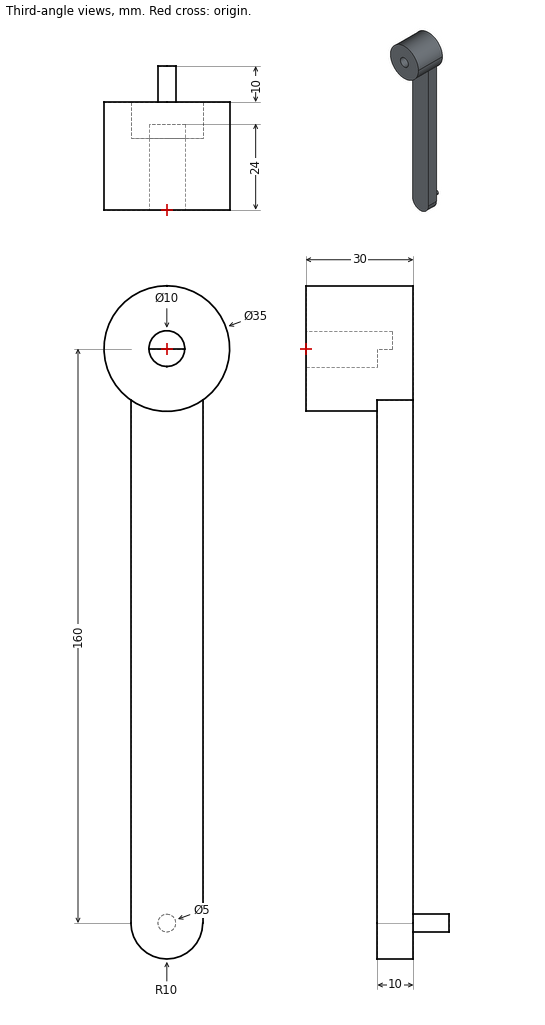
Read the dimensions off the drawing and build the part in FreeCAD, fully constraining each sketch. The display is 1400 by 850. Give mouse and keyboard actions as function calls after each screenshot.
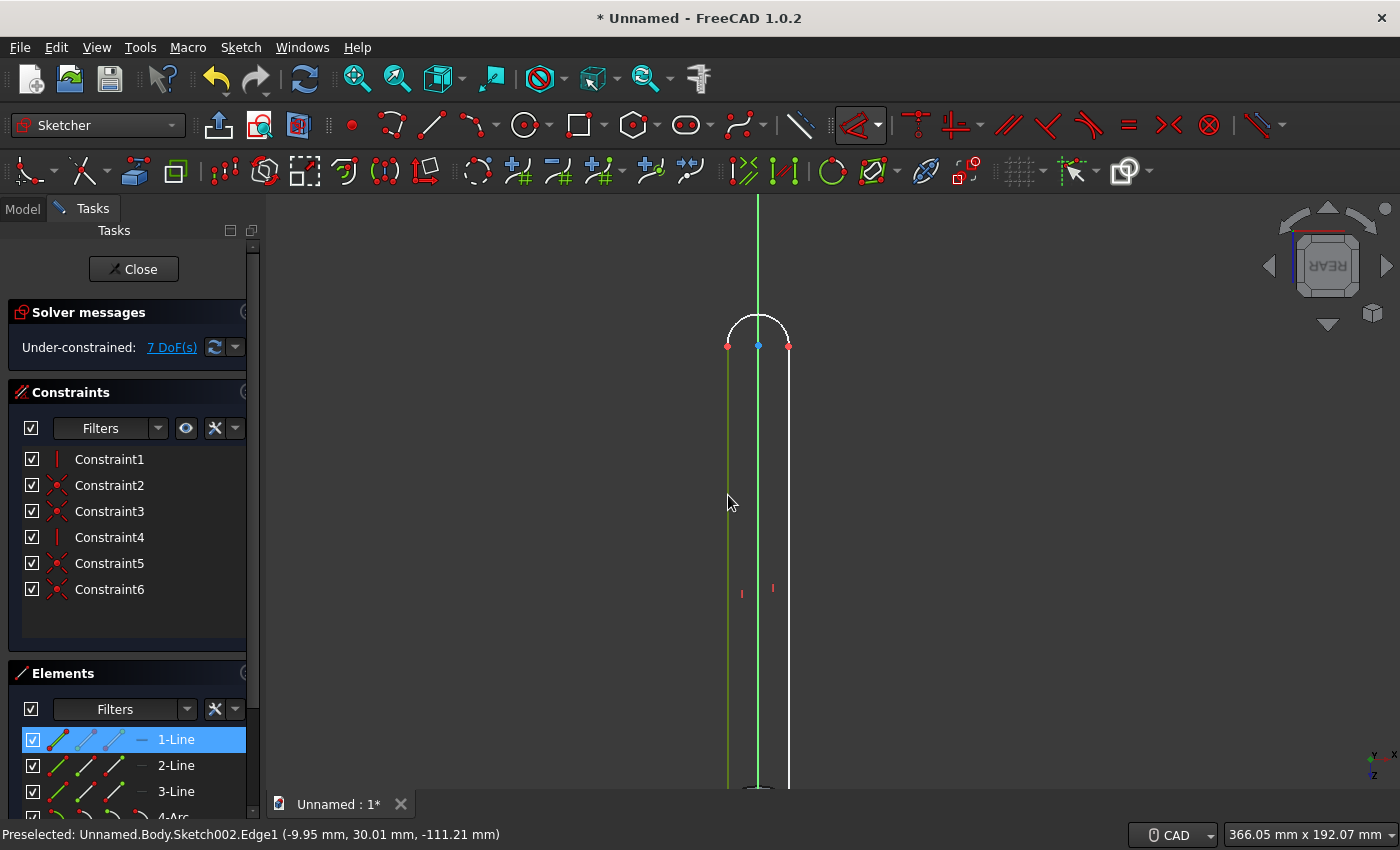
click(777, 321)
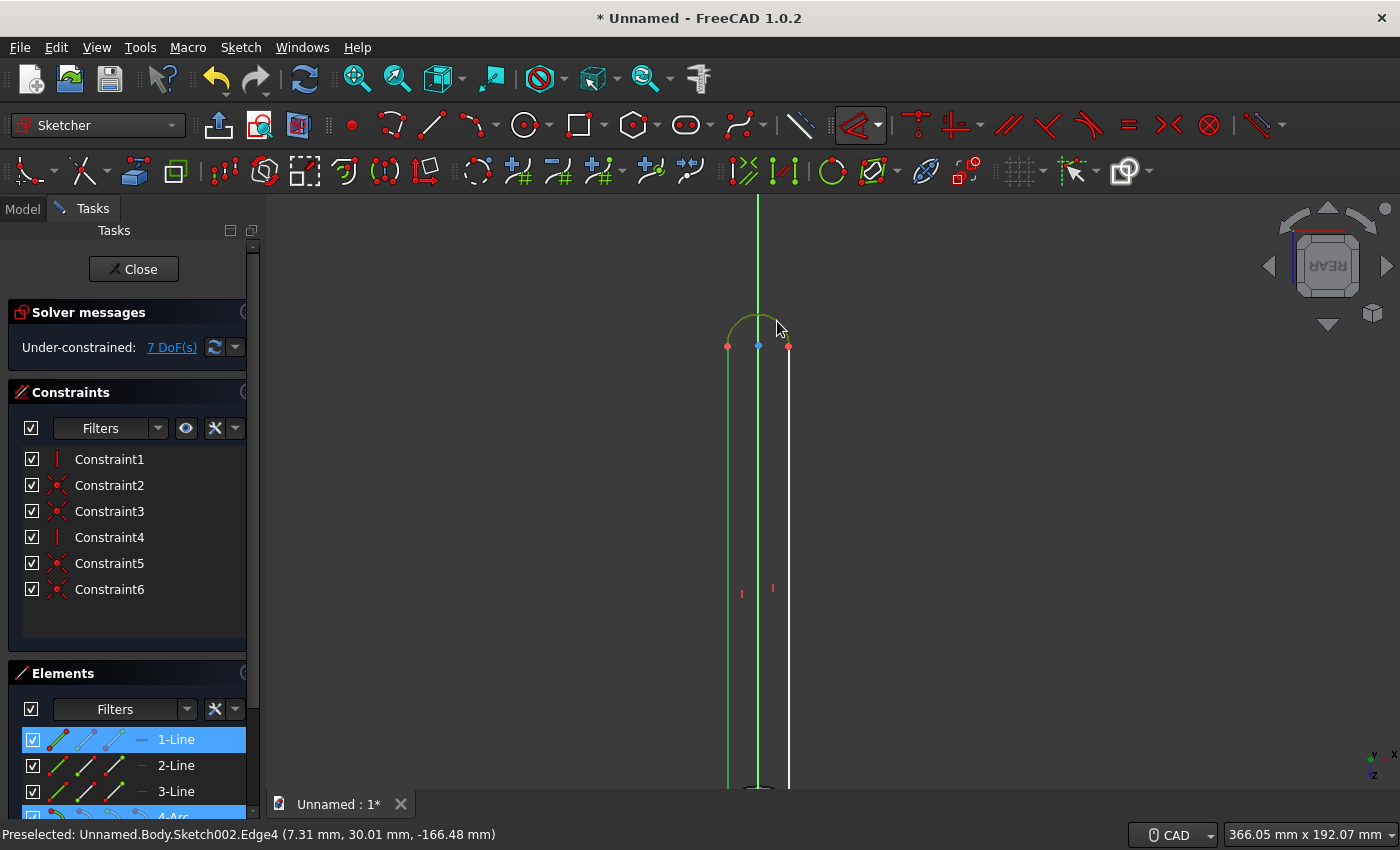
key(t)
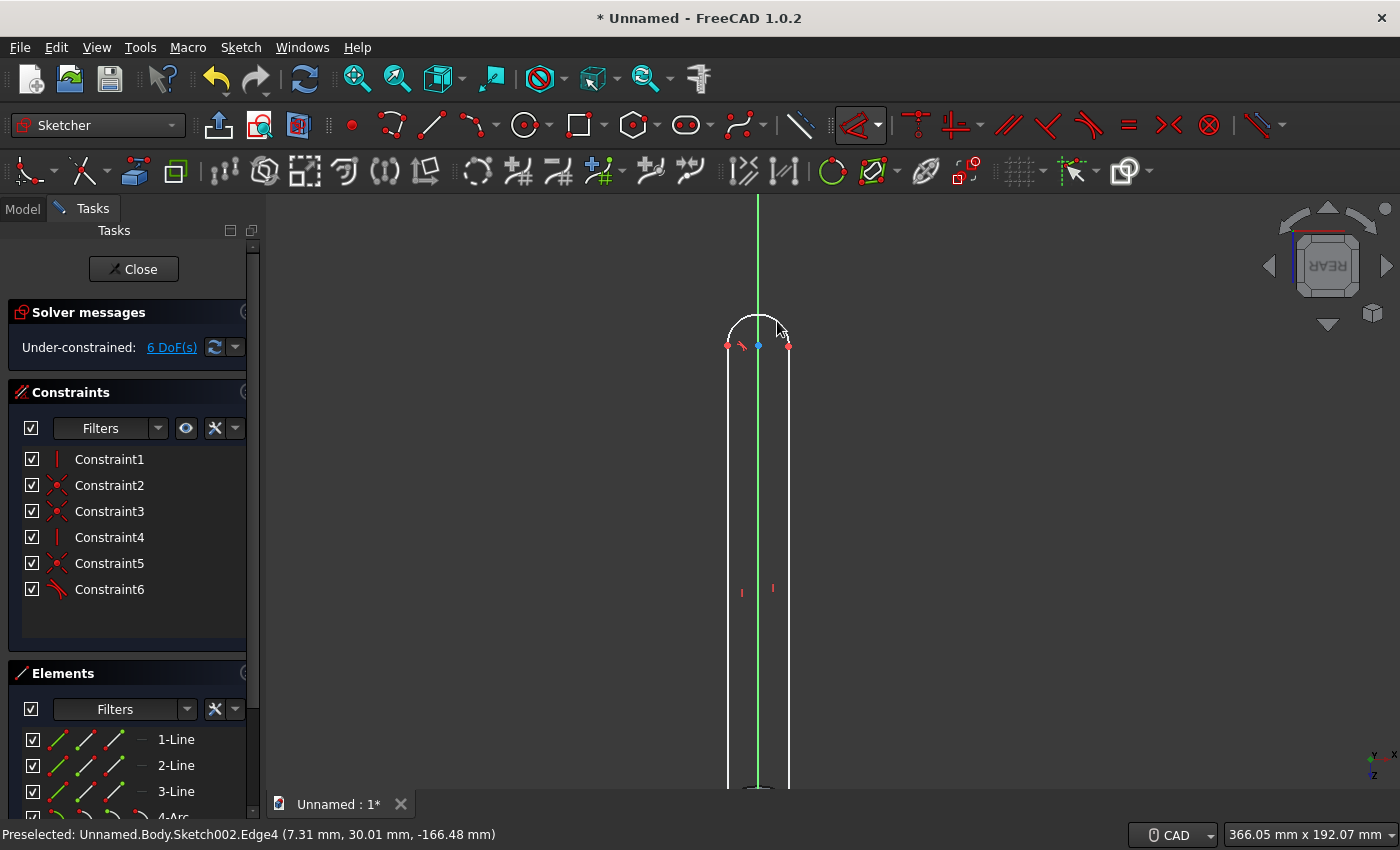
click(789, 684)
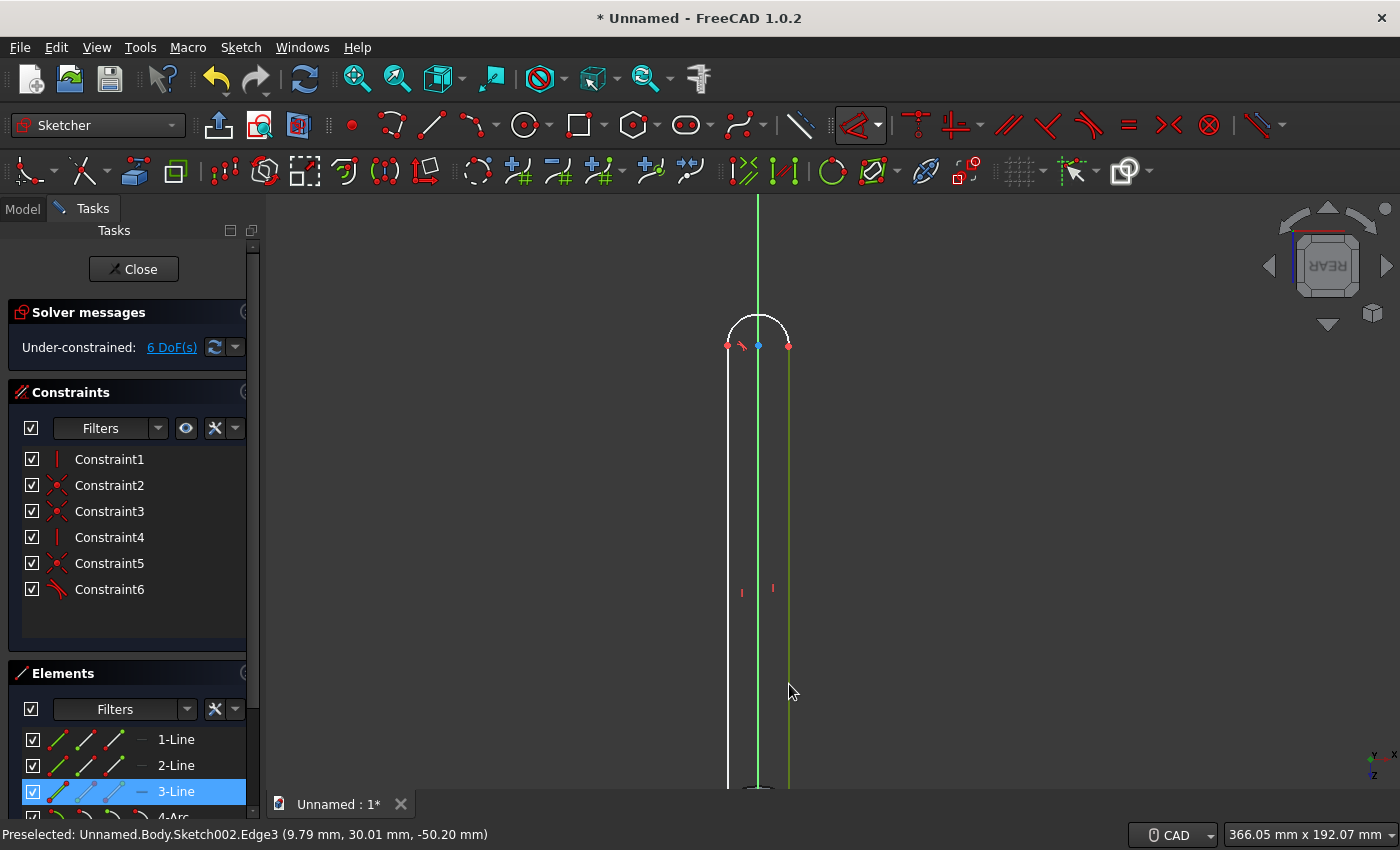
click(777, 321)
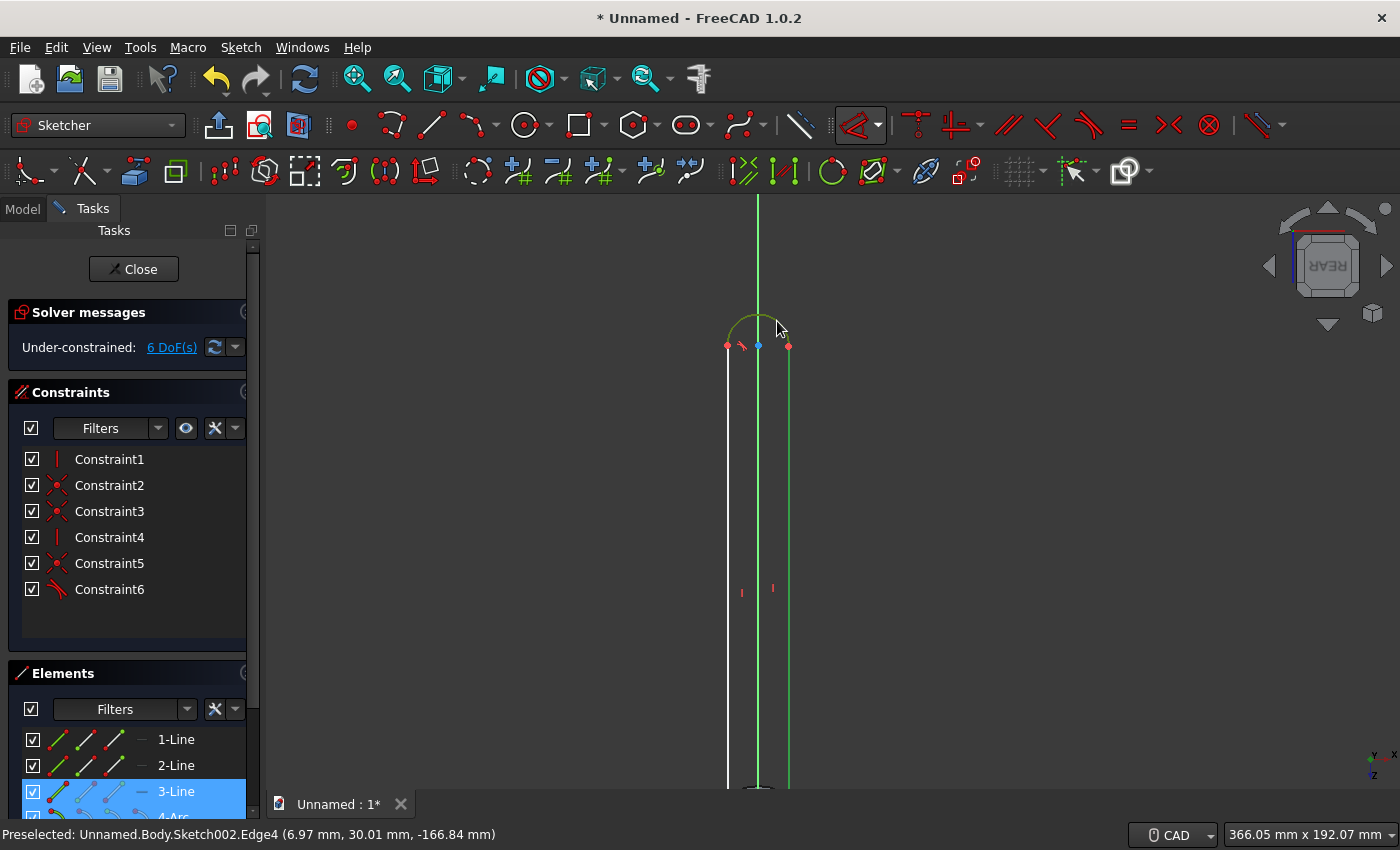
key(t)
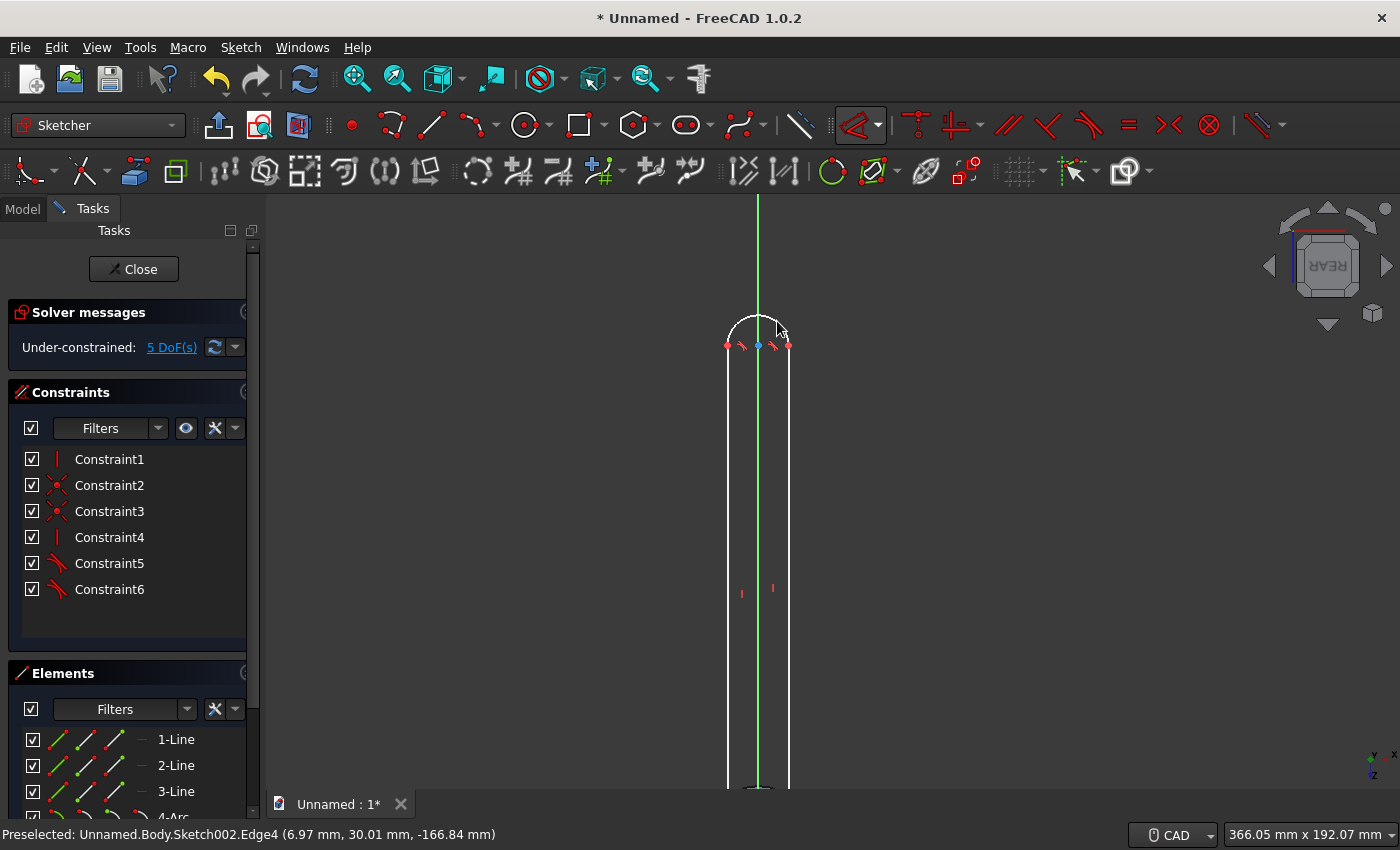
scroll(777, 317, down, 2)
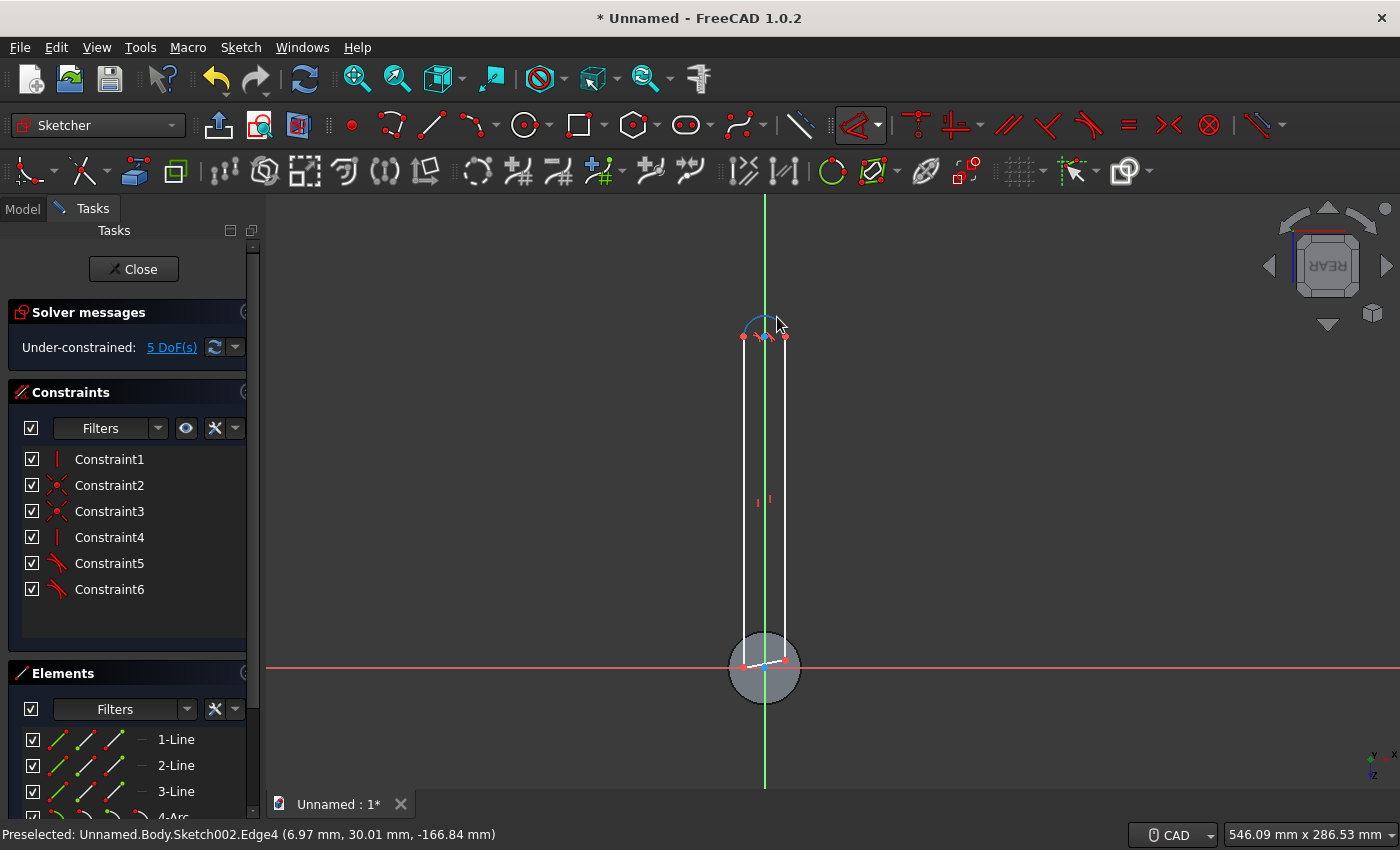
scroll(756, 666, up, 3)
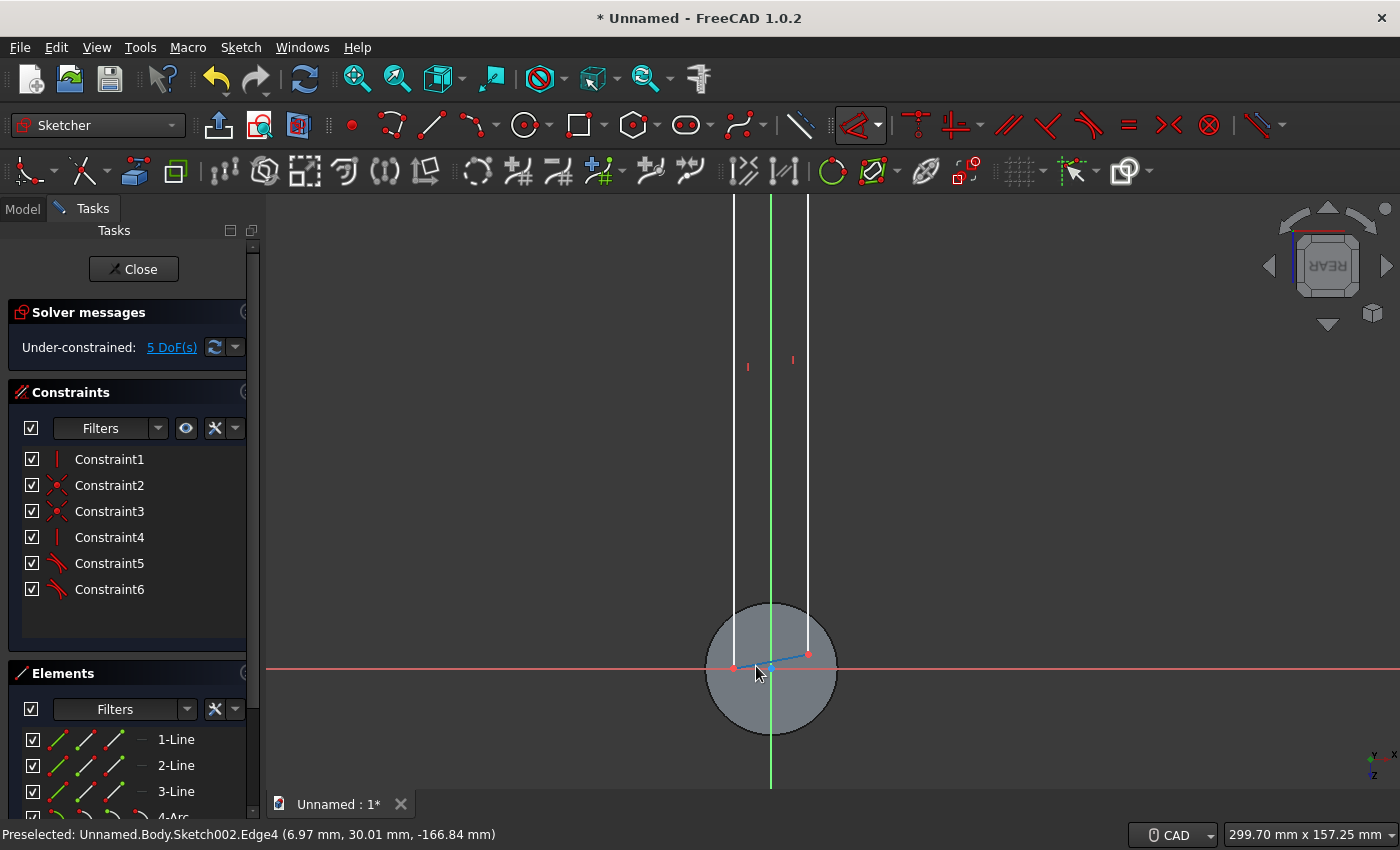
click(756, 665)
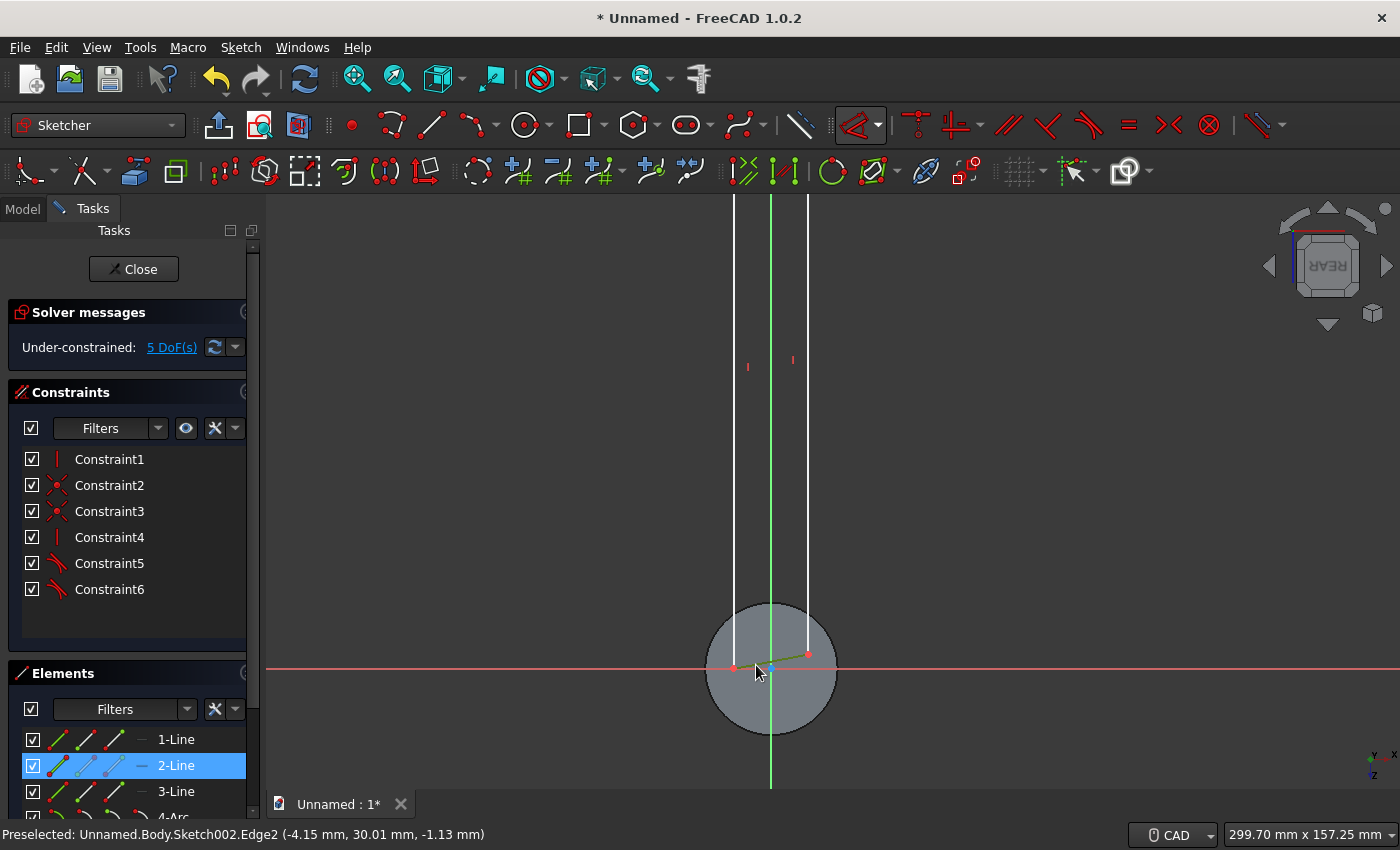
key(h)